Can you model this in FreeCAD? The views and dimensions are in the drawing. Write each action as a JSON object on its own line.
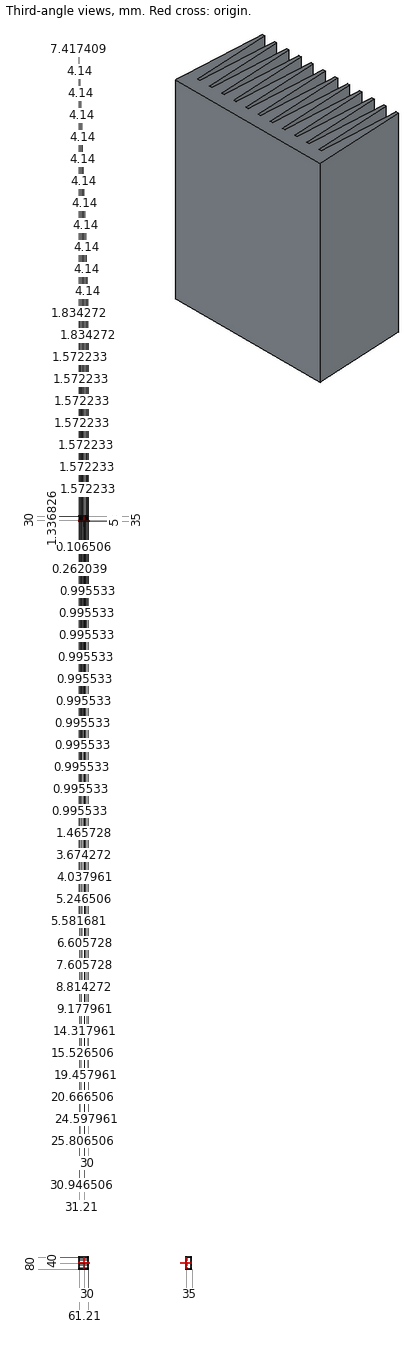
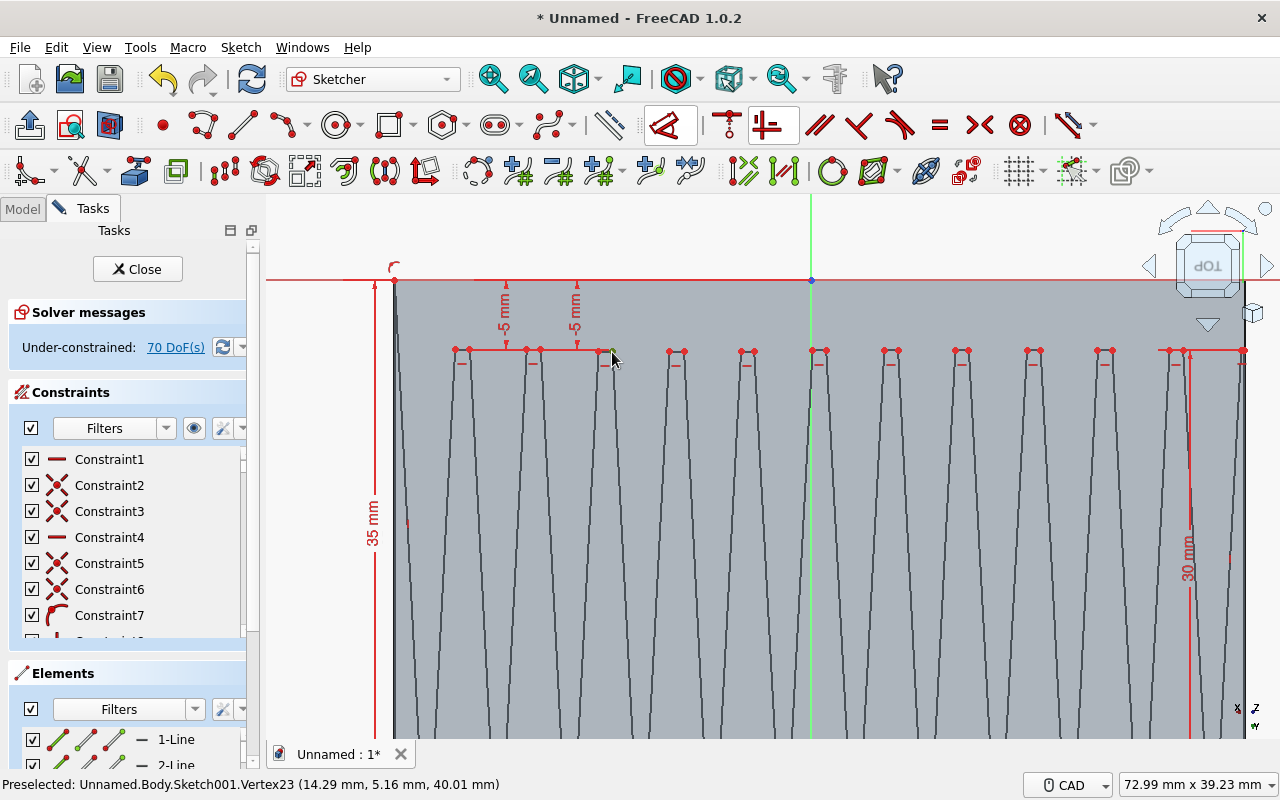
{"action": "left_click", "coordinate": [692, 126]}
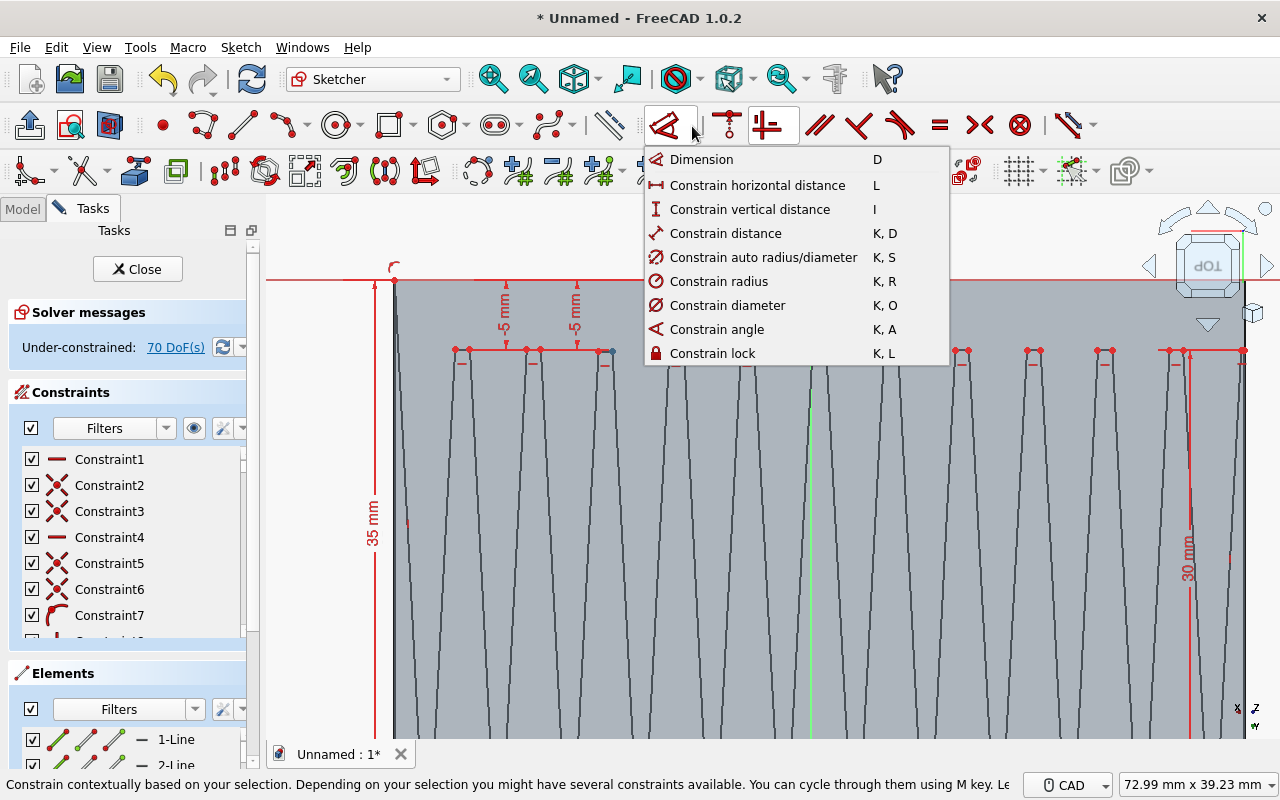
{"action": "left_click", "coordinate": [797, 209]}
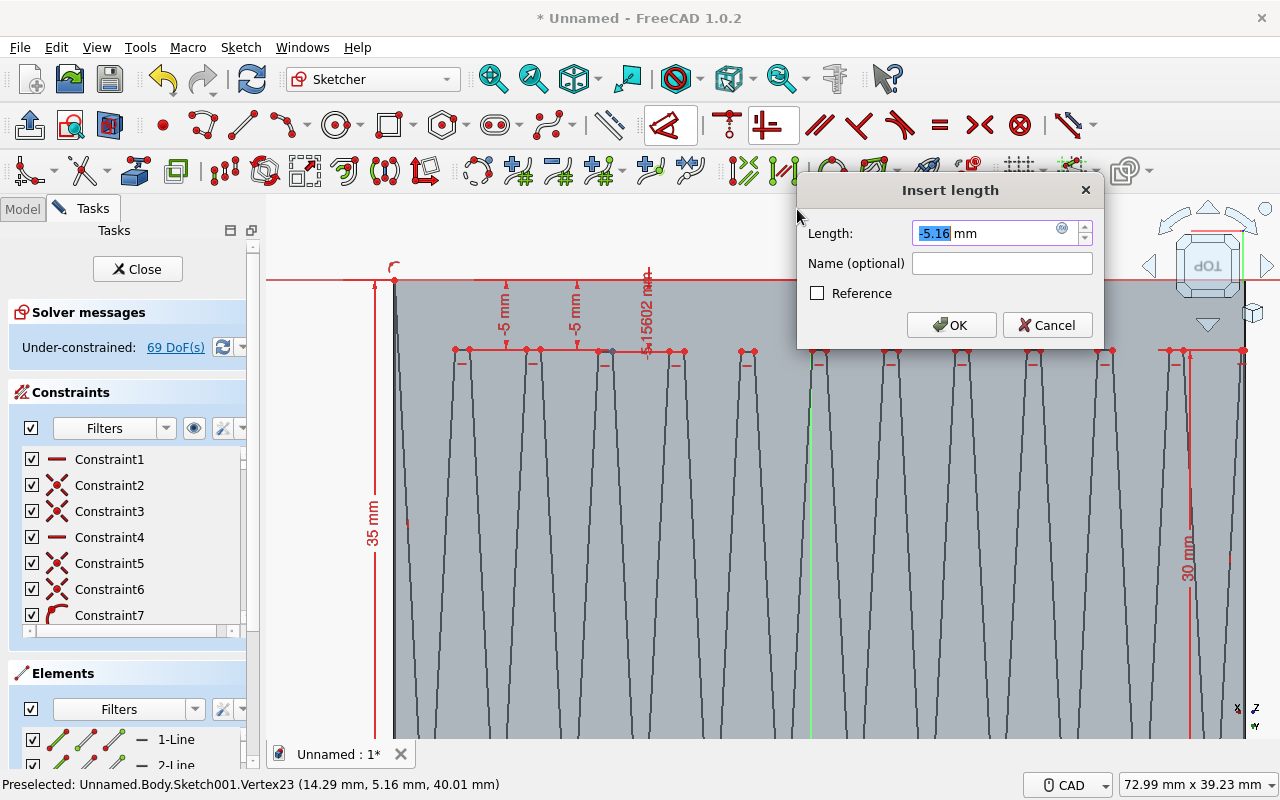
{"action": "type", "text": "-5"}
{"action": "key", "text": "Return"}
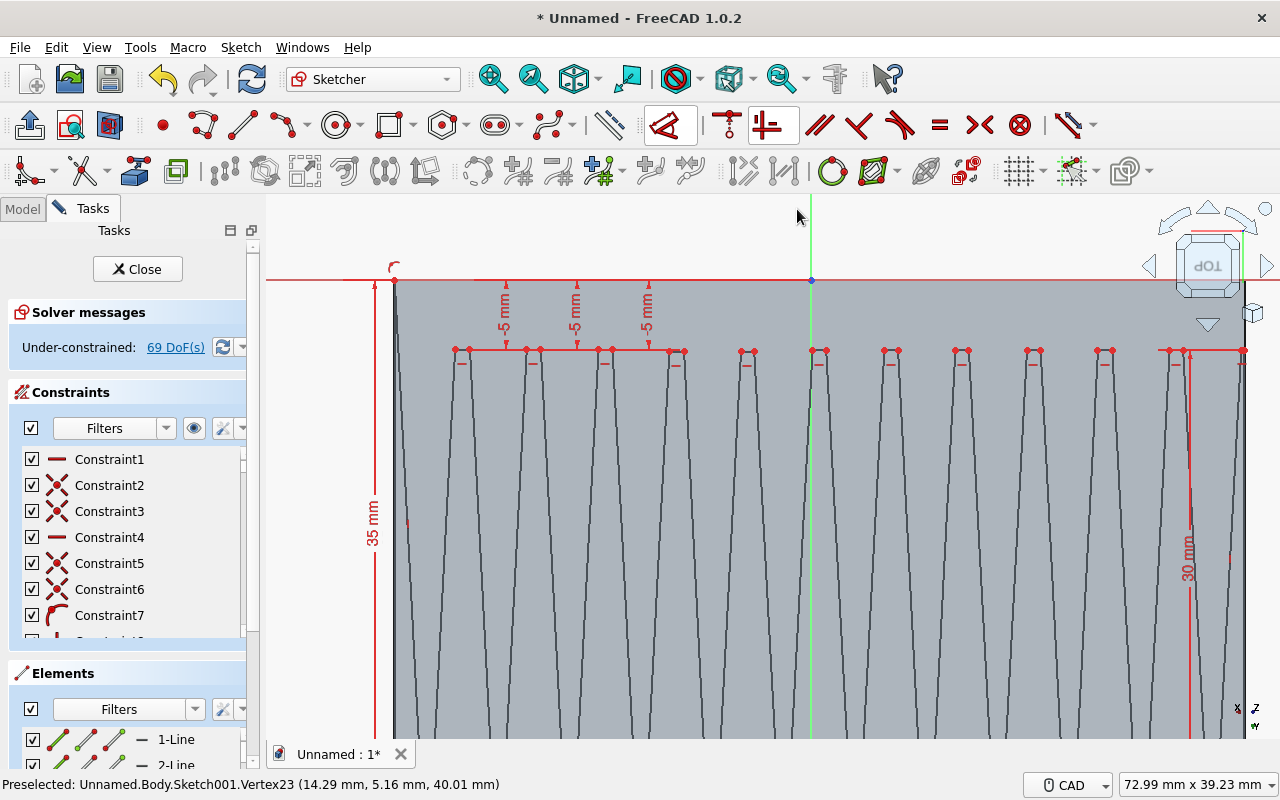
{"action": "left_click", "coordinate": [684, 352]}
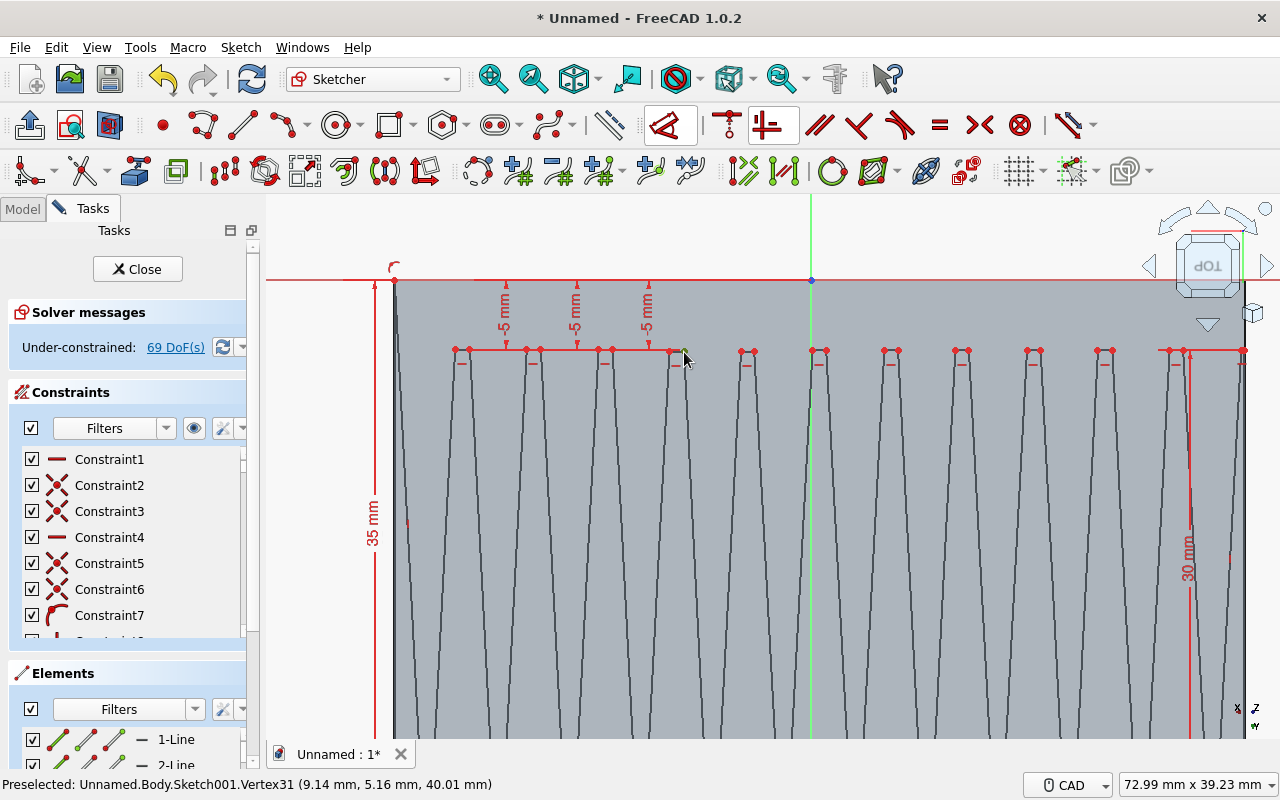
{"action": "left_click", "coordinate": [692, 126]}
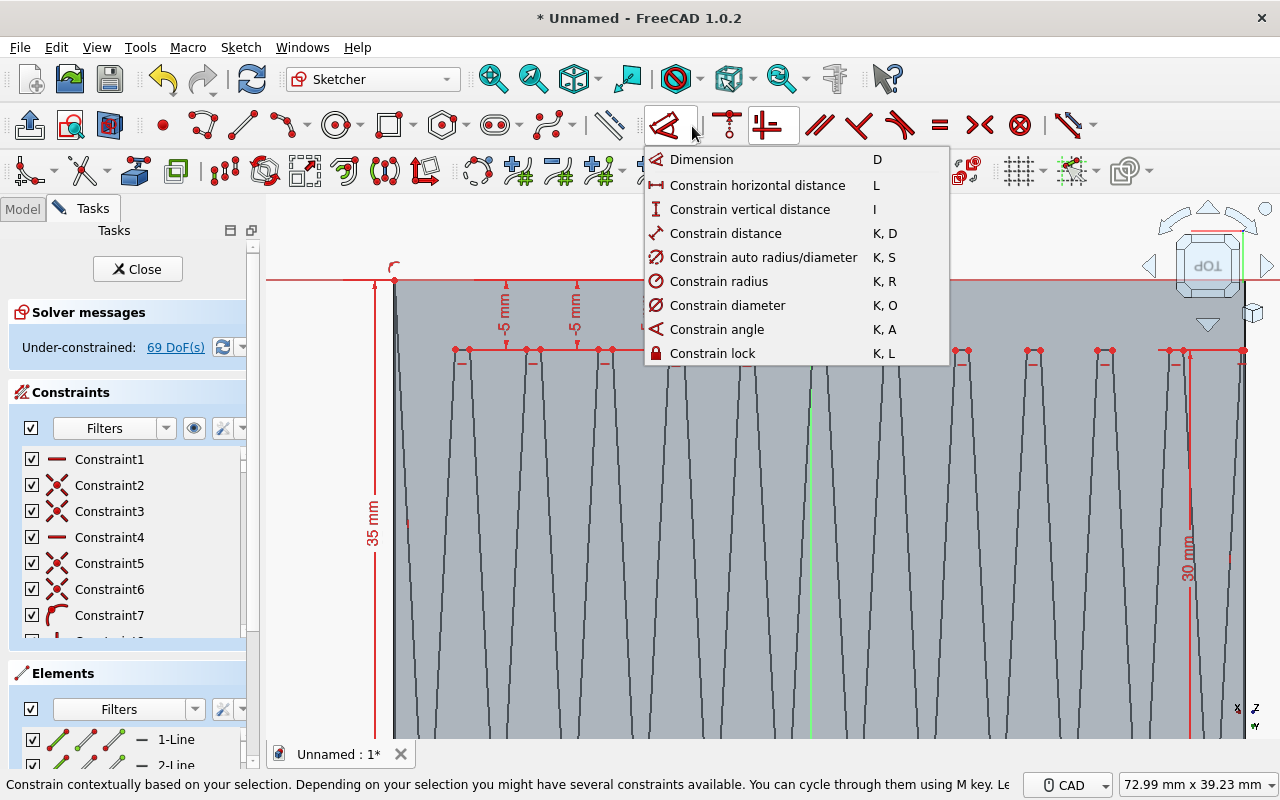
{"action": "left_click", "coordinate": [797, 209]}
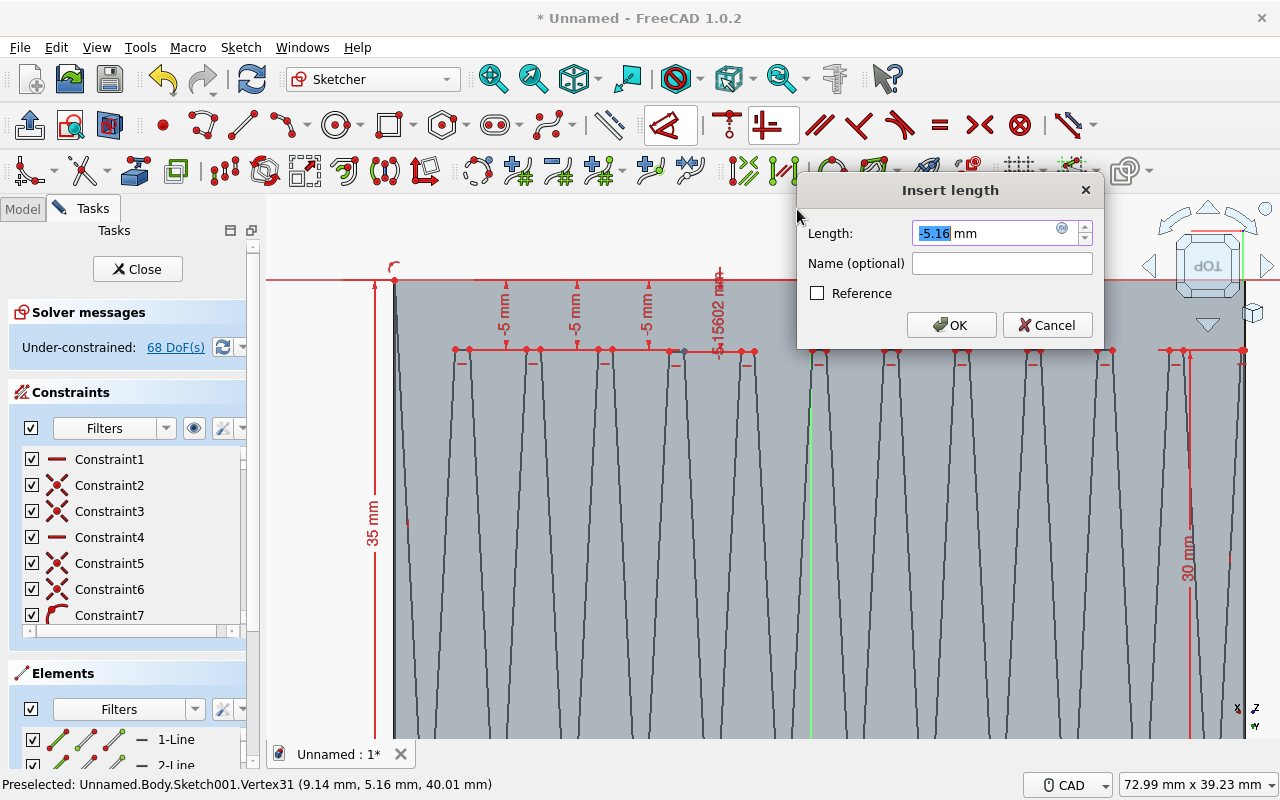
{"action": "type", "text": "-5"}
{"action": "key", "text": "Return"}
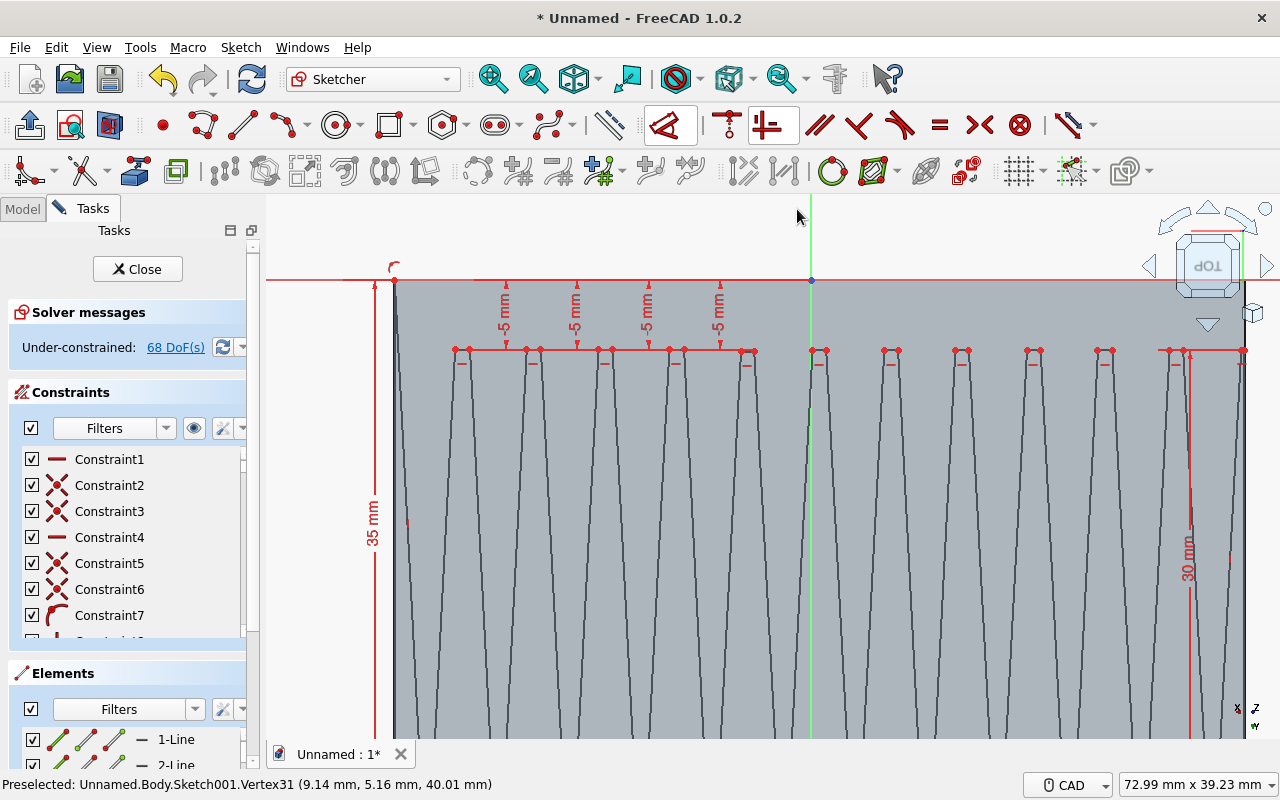
{"action": "left_click", "coordinate": [754, 352]}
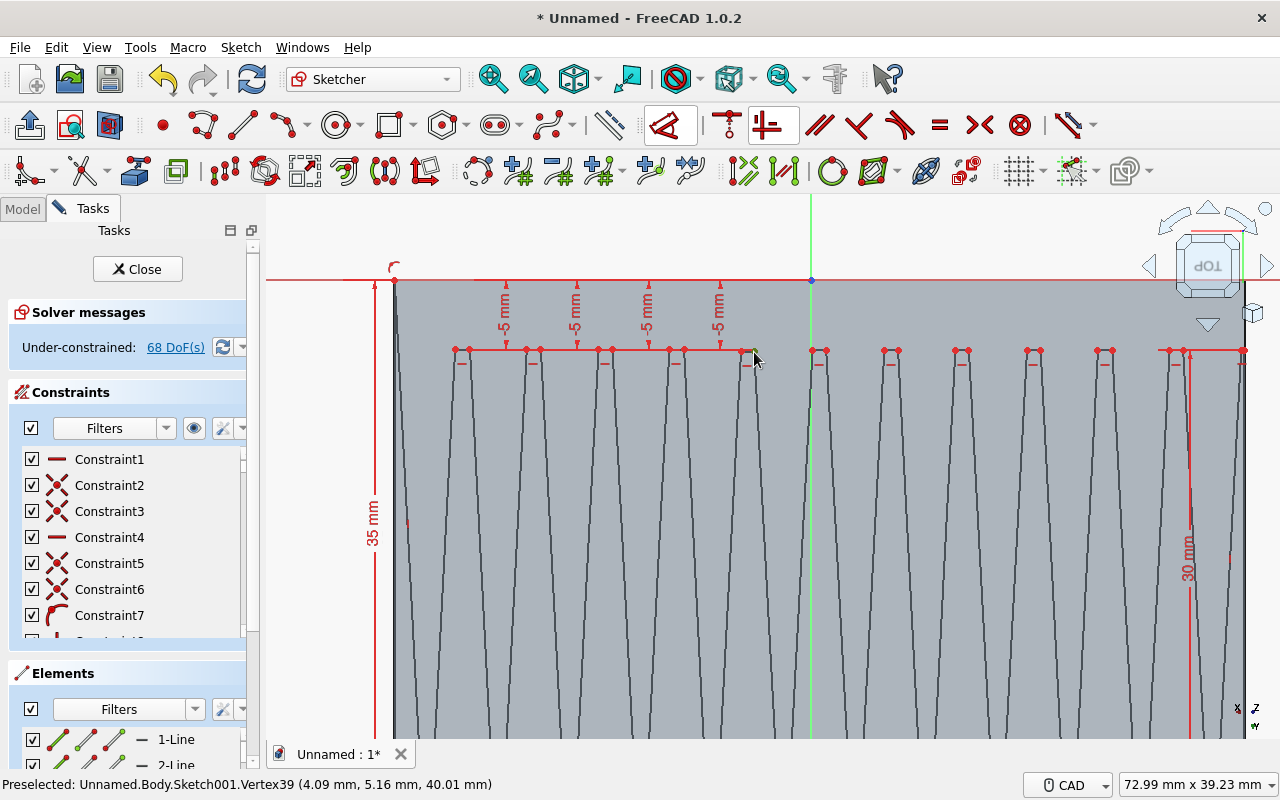
{"action": "key", "text": "i"}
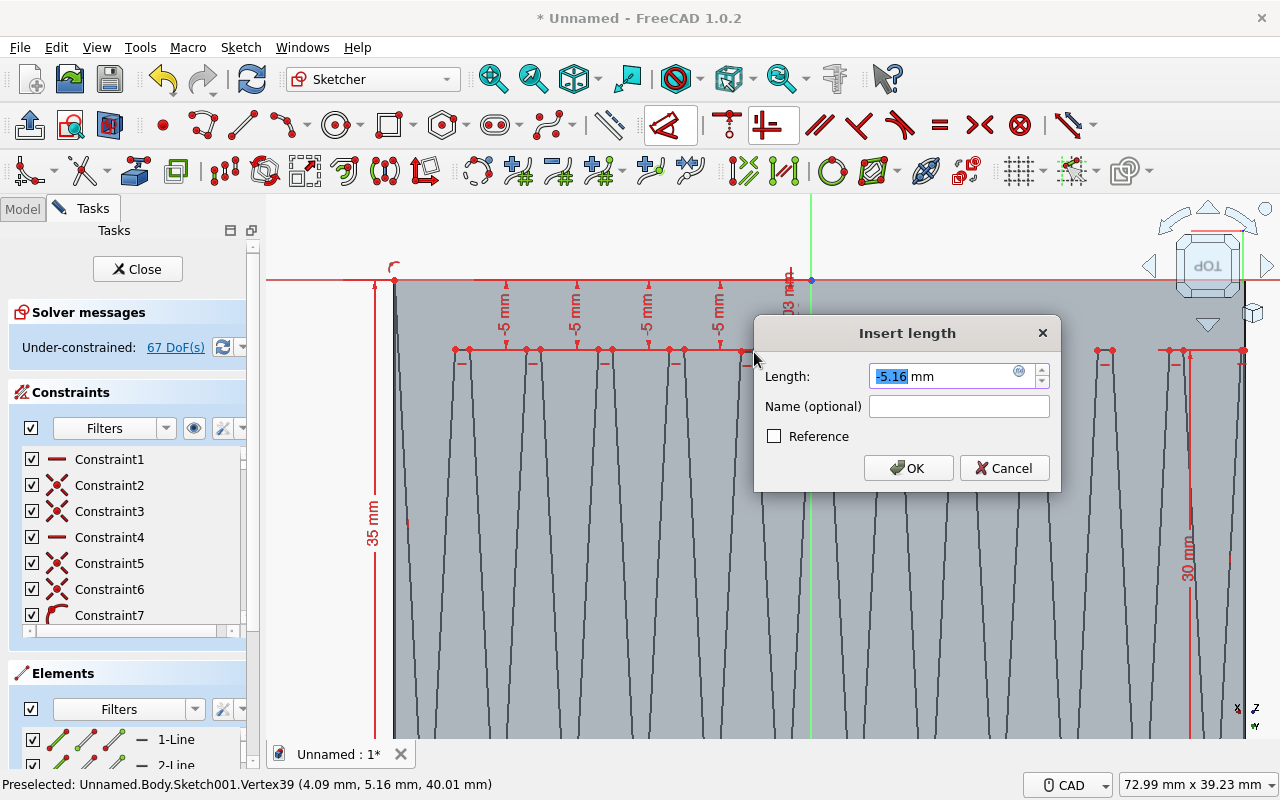
{"action": "type", "text": "-5"}
{"action": "key", "text": "Return"}